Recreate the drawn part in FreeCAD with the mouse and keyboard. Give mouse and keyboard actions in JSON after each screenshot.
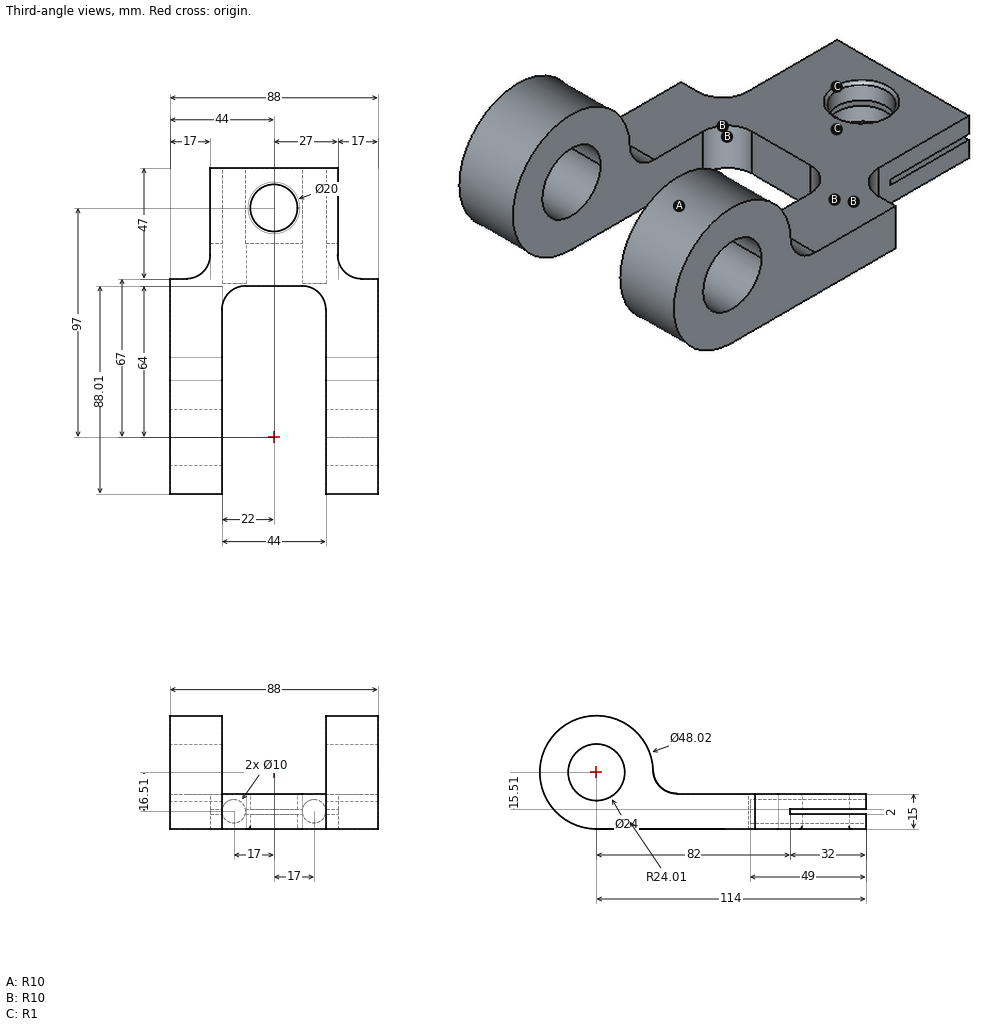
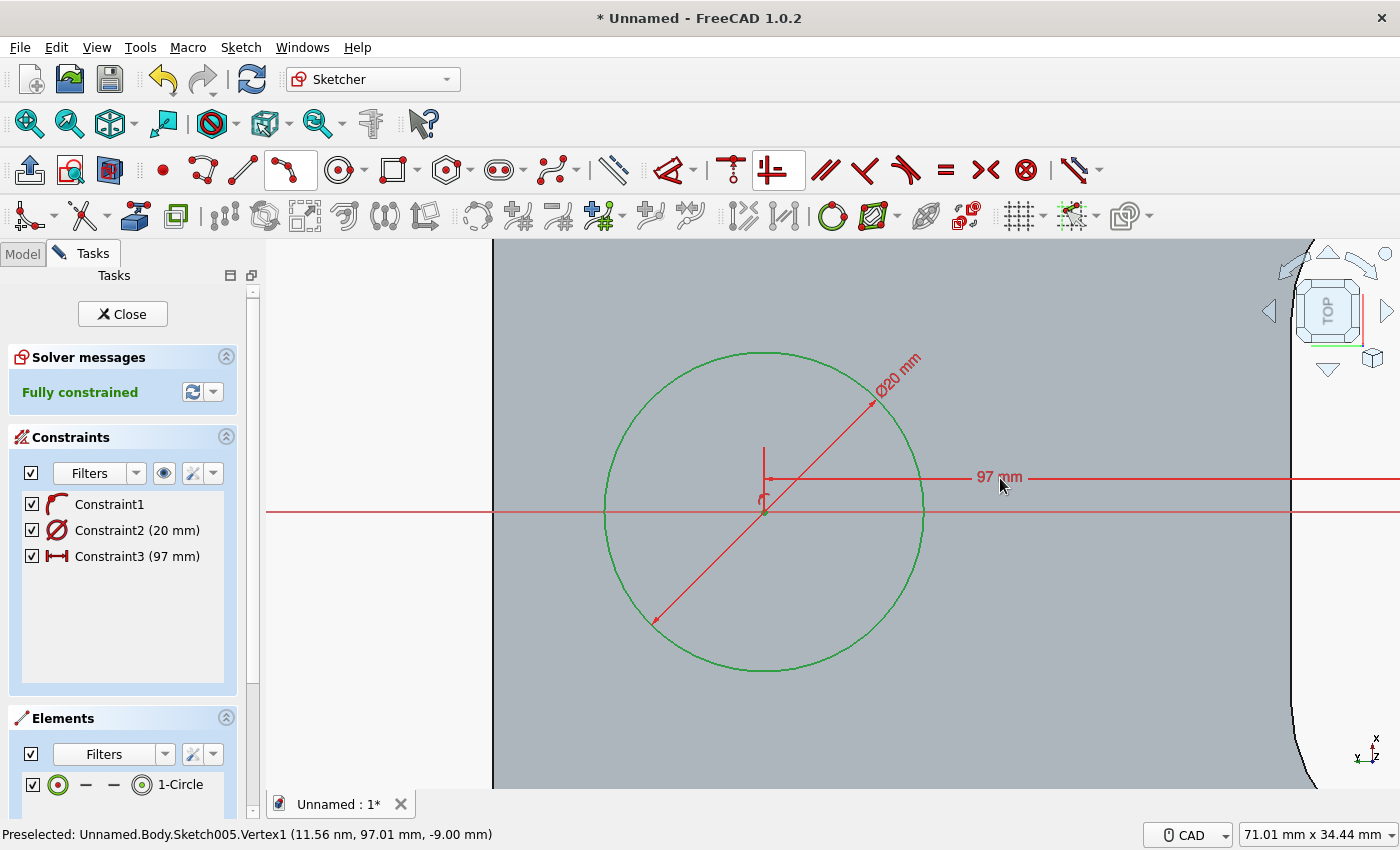
{"action": "left_click", "coordinate": [123, 314]}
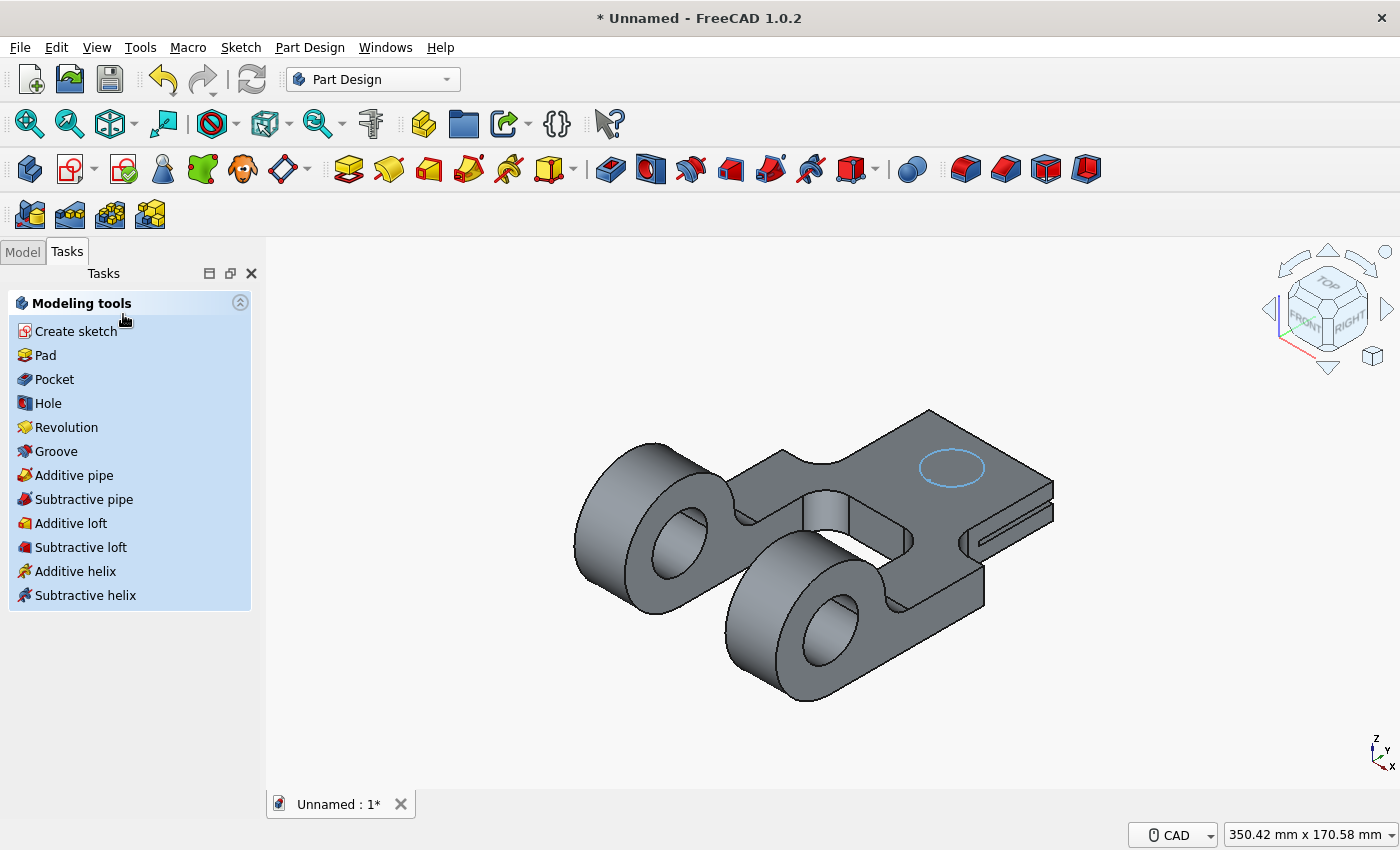
{"action": "left_click", "coordinate": [612, 170]}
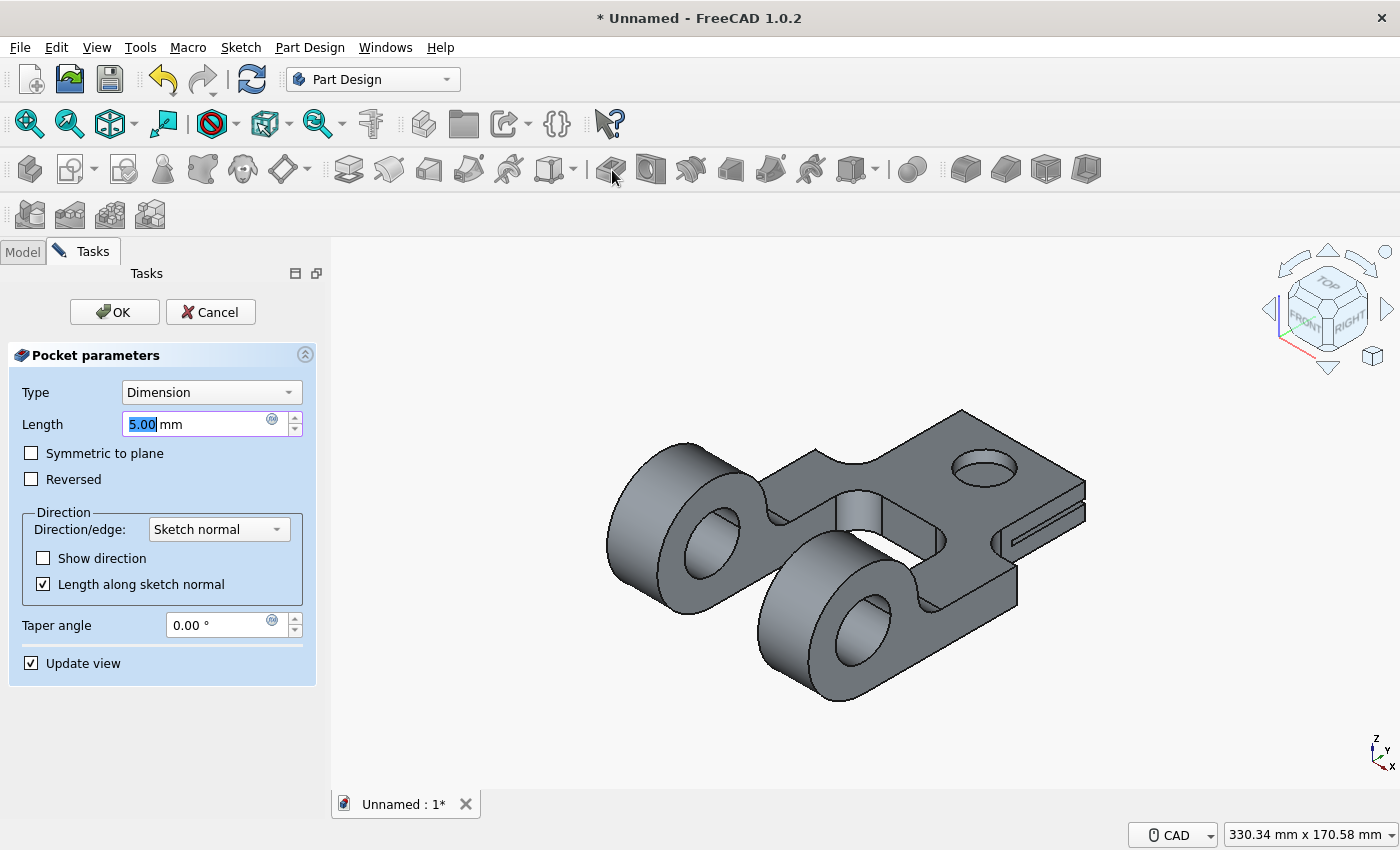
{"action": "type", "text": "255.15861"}
{"action": "key", "text": "Tab"}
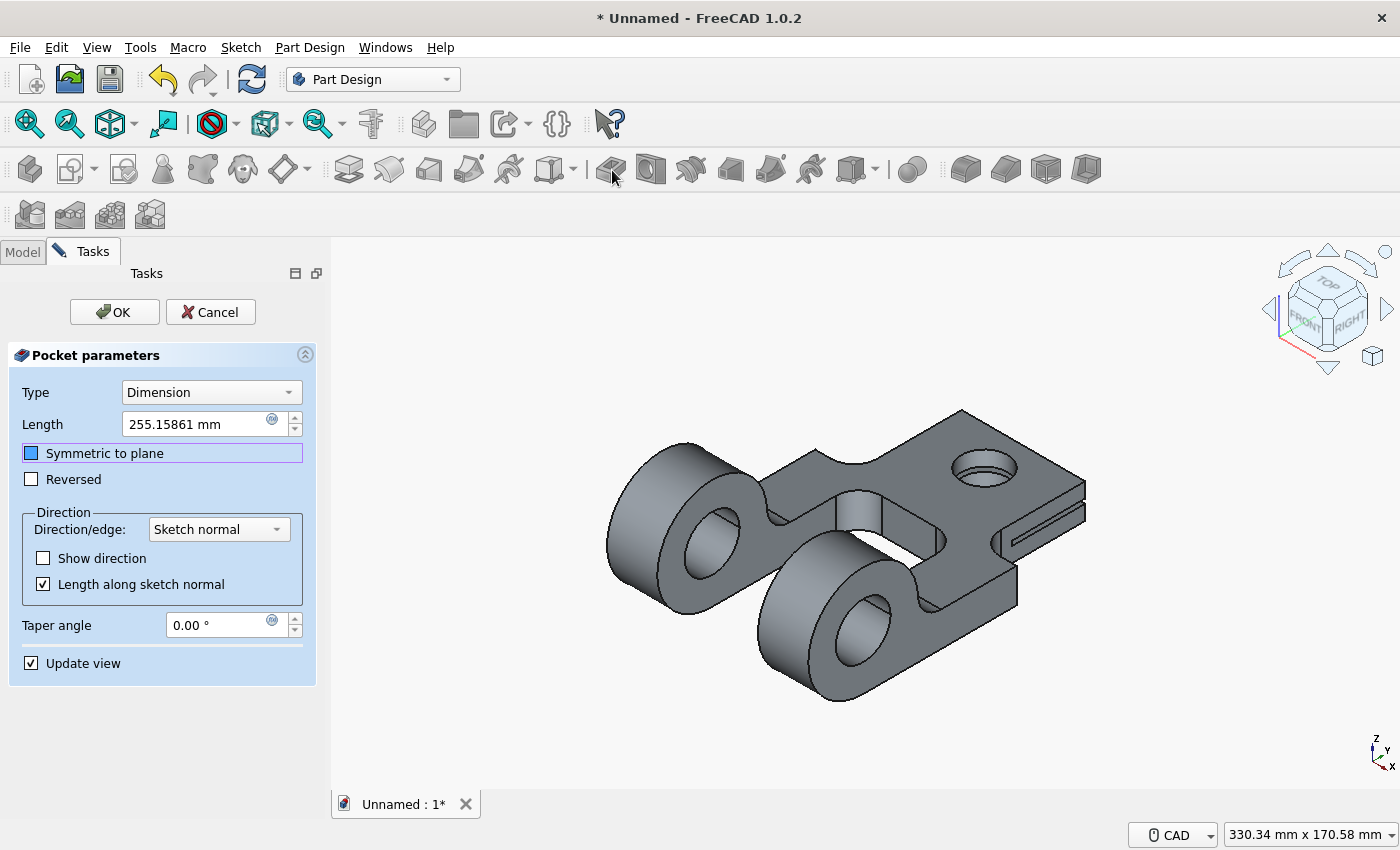
{"action": "left_click", "coordinate": [30, 453]}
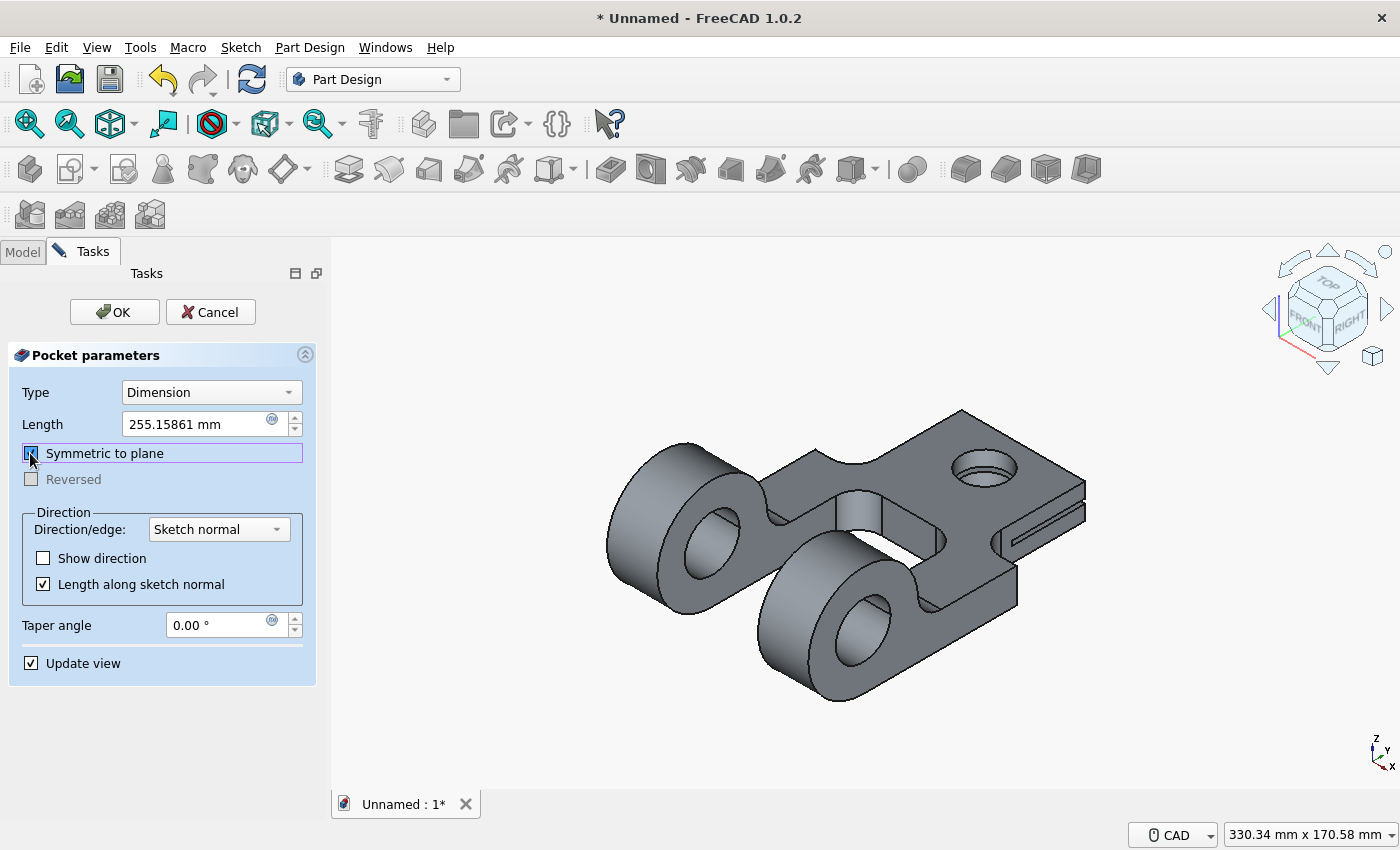
{"action": "left_click", "coordinate": [115, 312]}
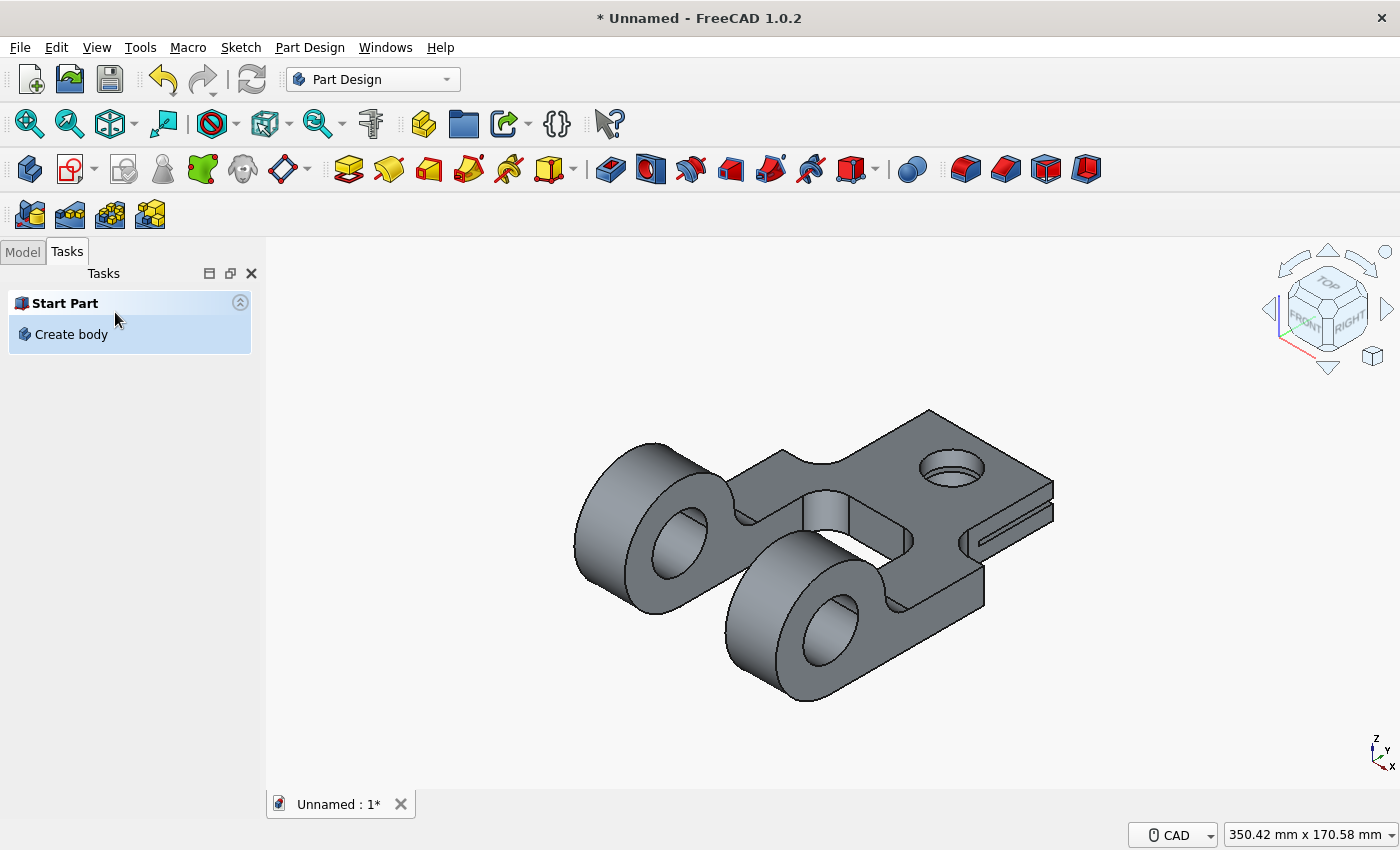
{"action": "left_click", "coordinate": [975, 454]}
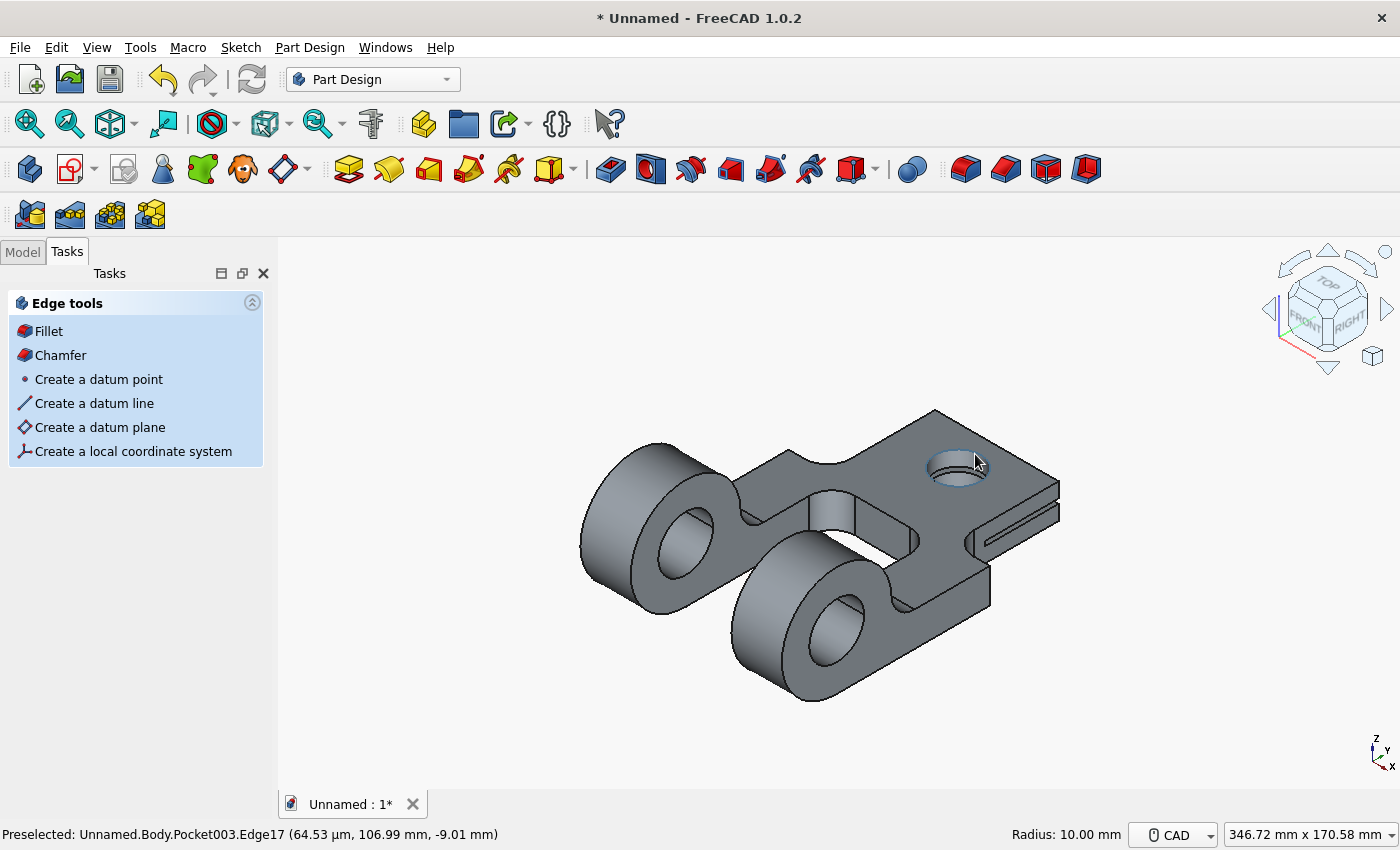
{"action": "key", "text": "2"}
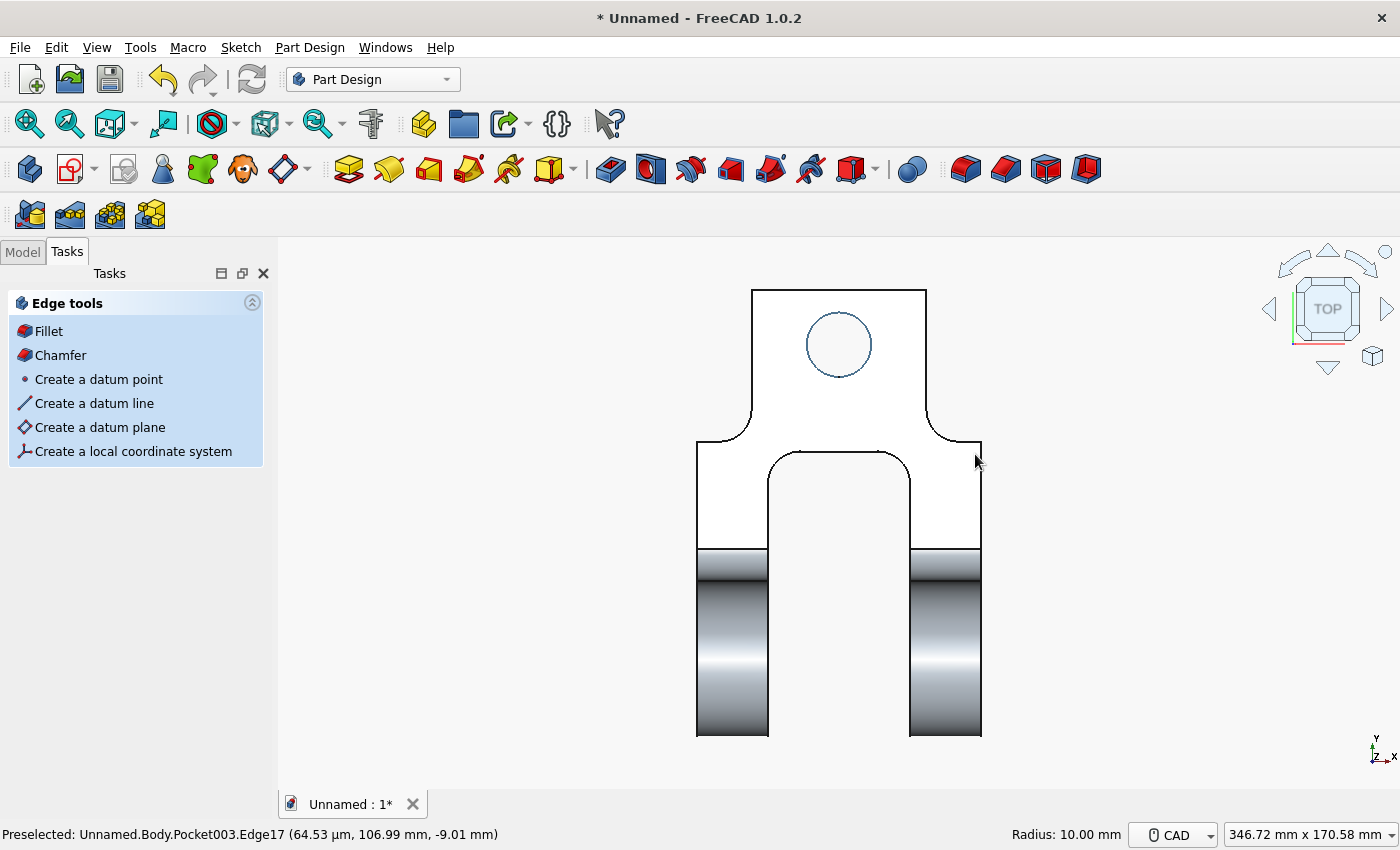
{"action": "key", "text": "0"}